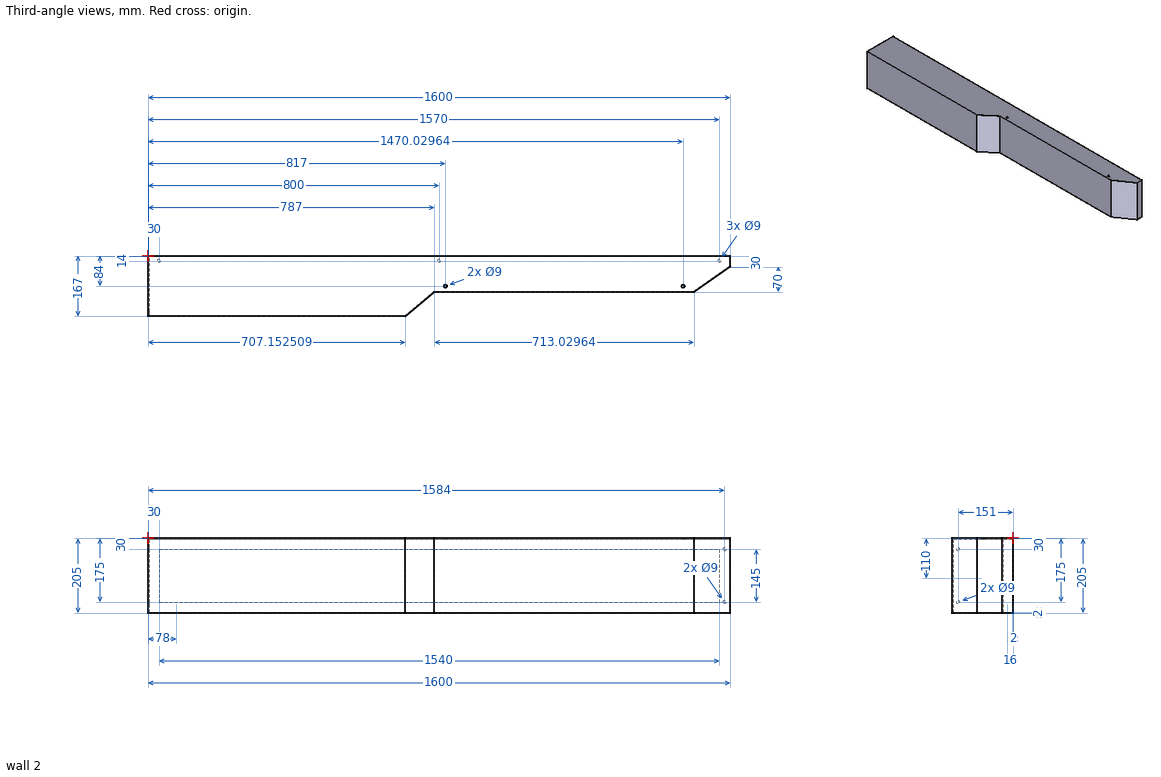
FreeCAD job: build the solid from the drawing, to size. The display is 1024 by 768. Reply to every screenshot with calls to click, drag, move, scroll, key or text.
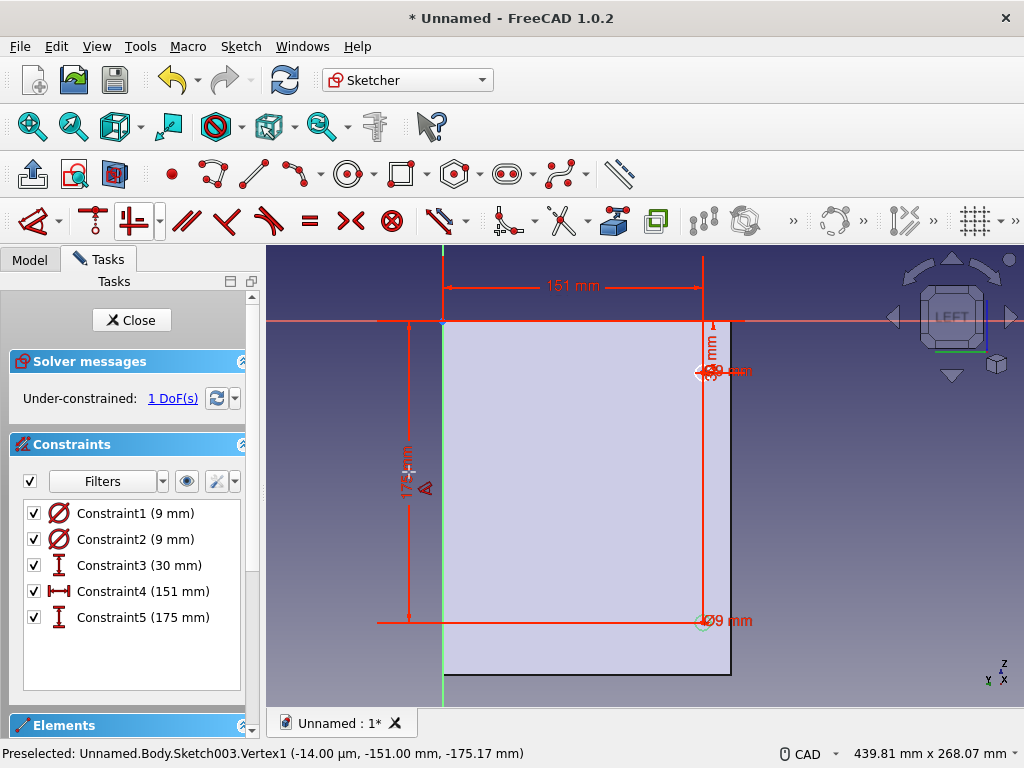
click(703, 373)
click(482, 287)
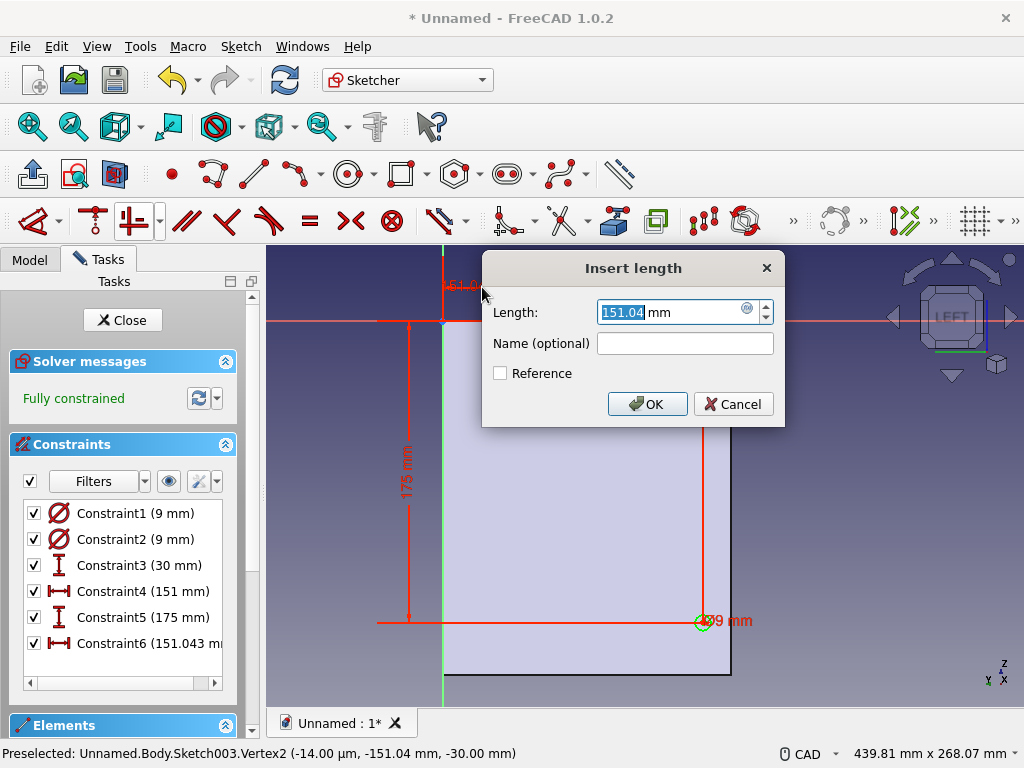
text(151)
key(Return)
key(Escape)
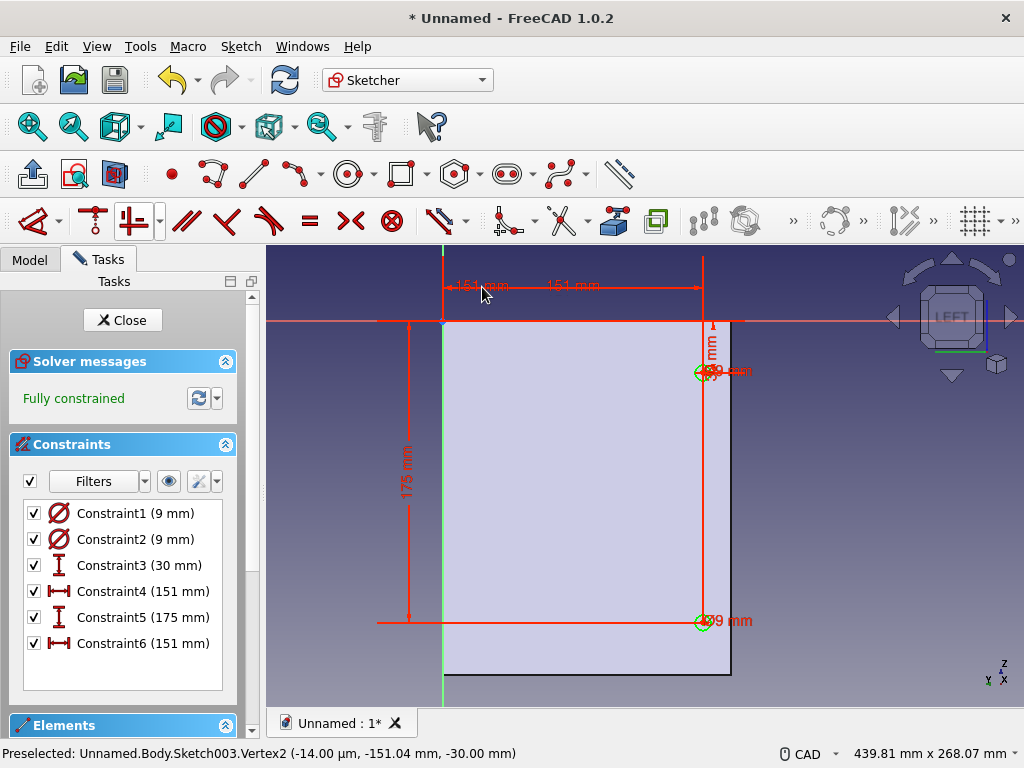
click(123, 320)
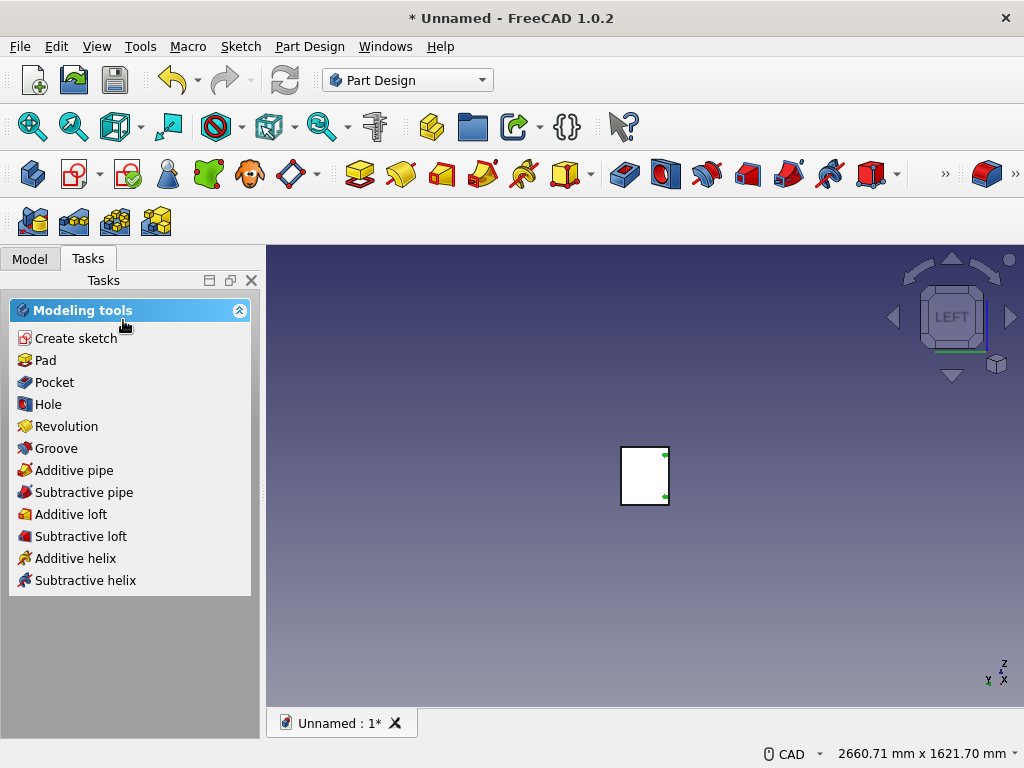
click(625, 174)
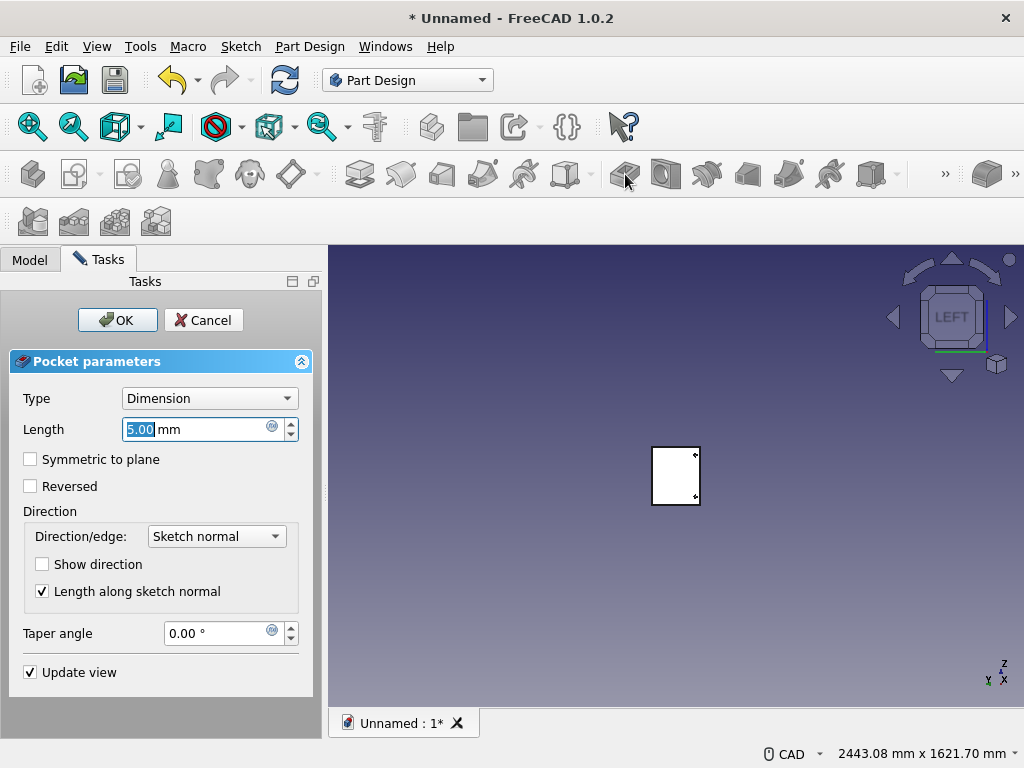
text(78)
key(Tab)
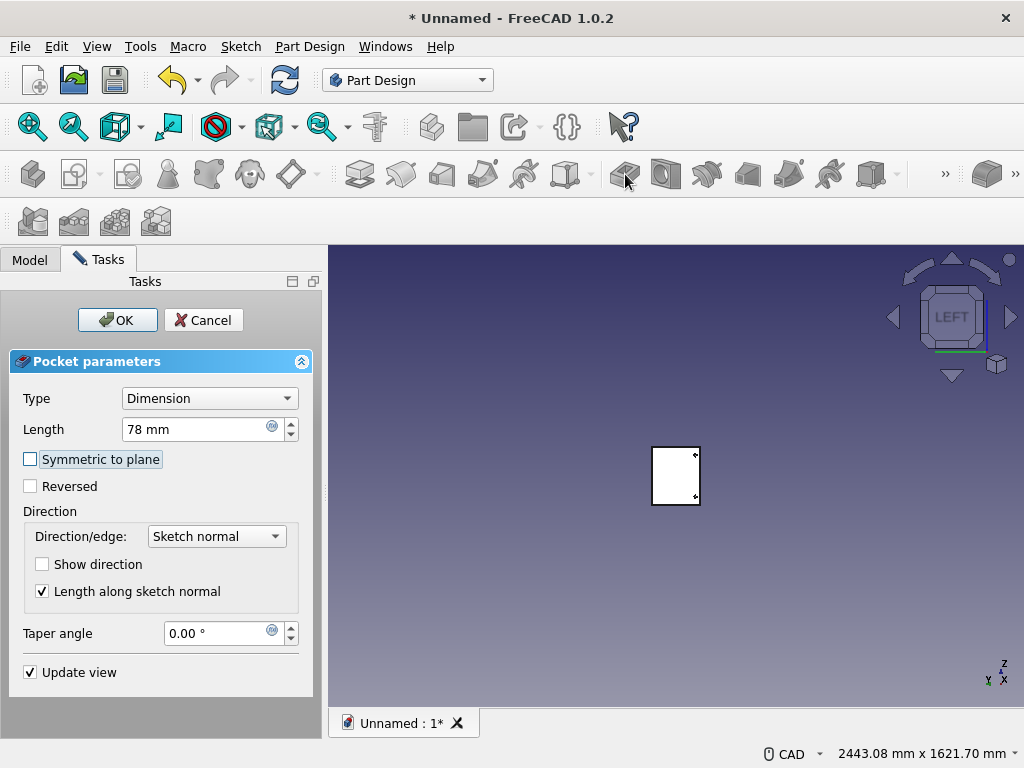
click(118, 320)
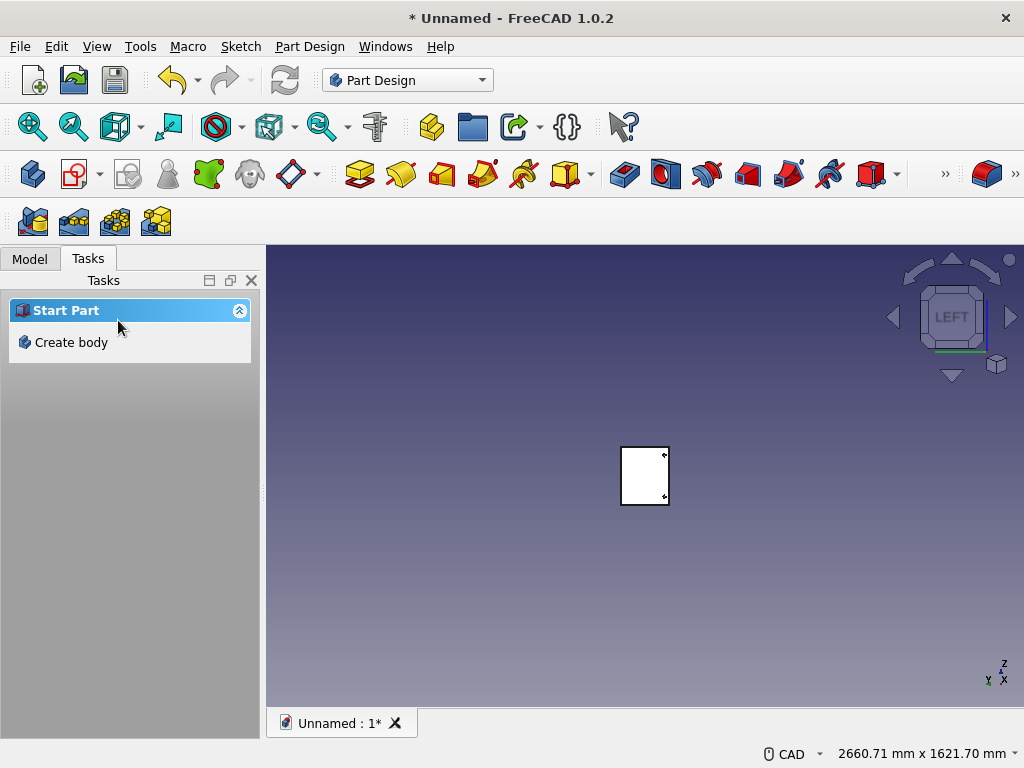
key(v)
key(f)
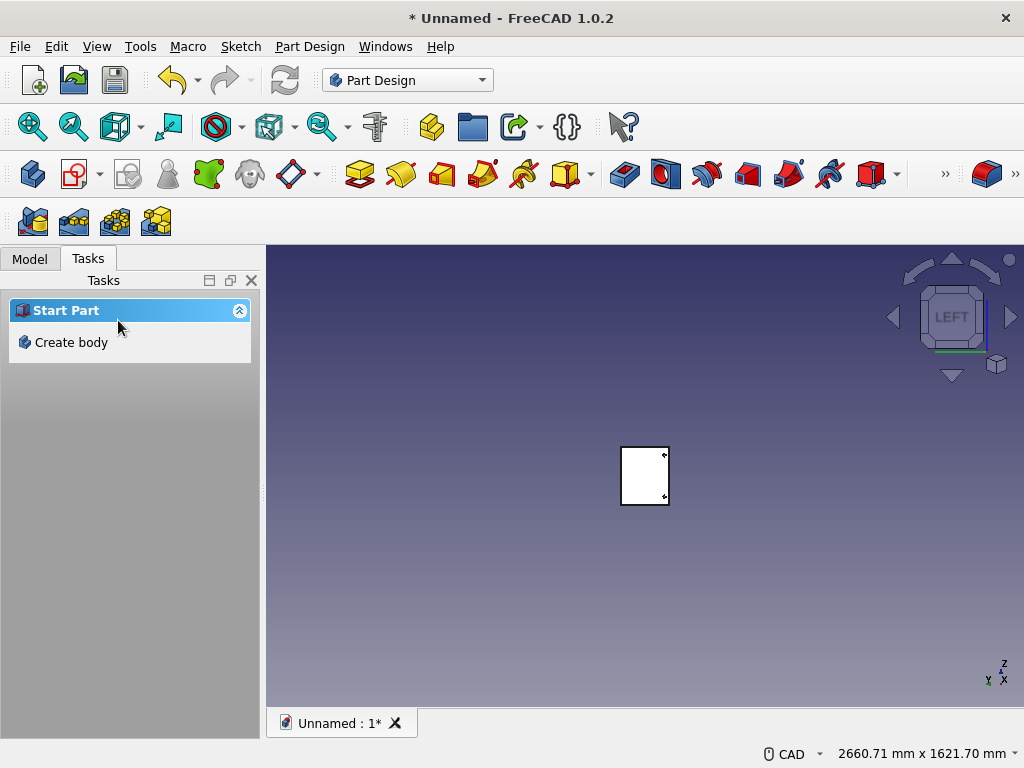
key(4)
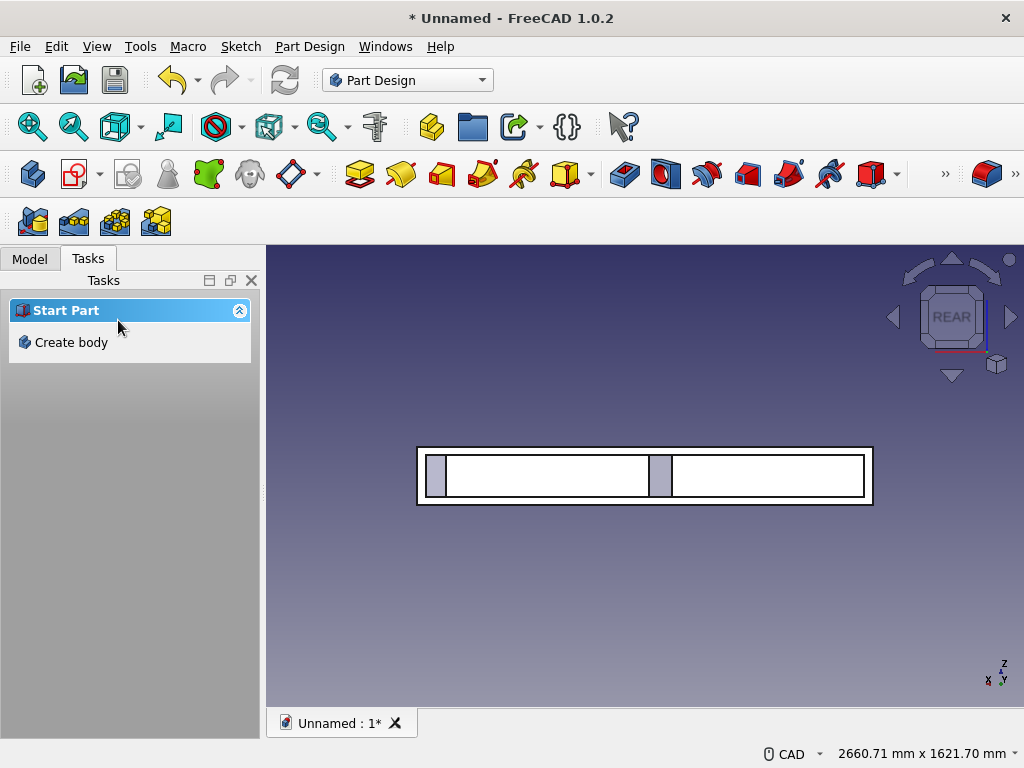
scroll(450, 450, up, 6)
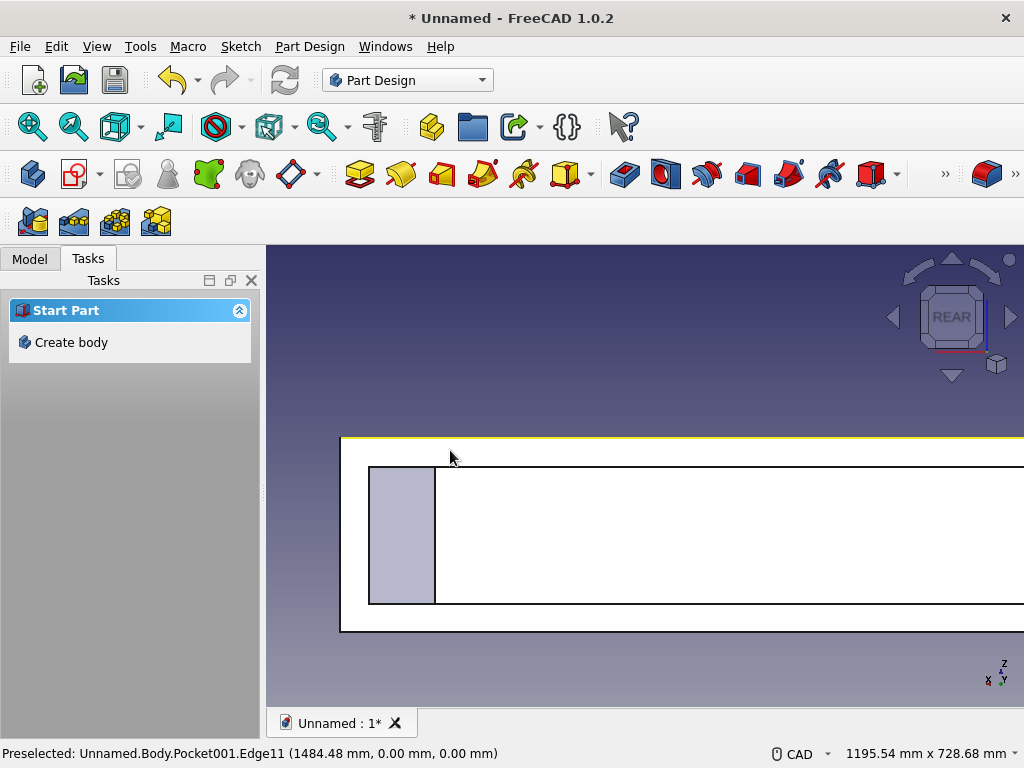
click(448, 451)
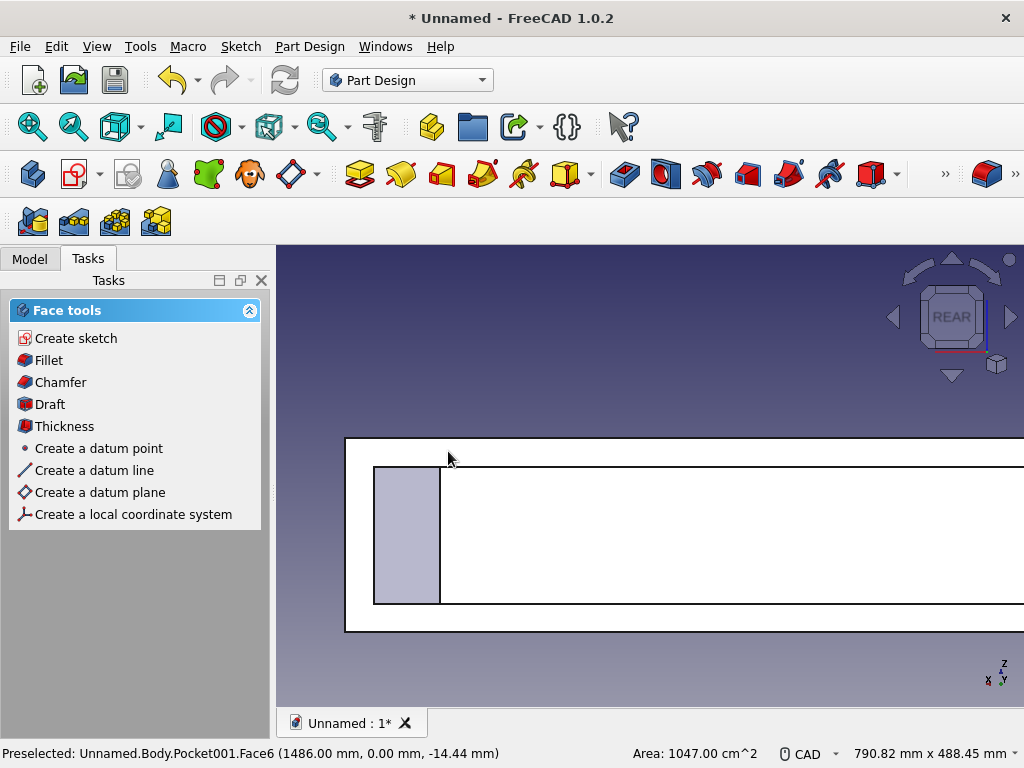
click(74, 174)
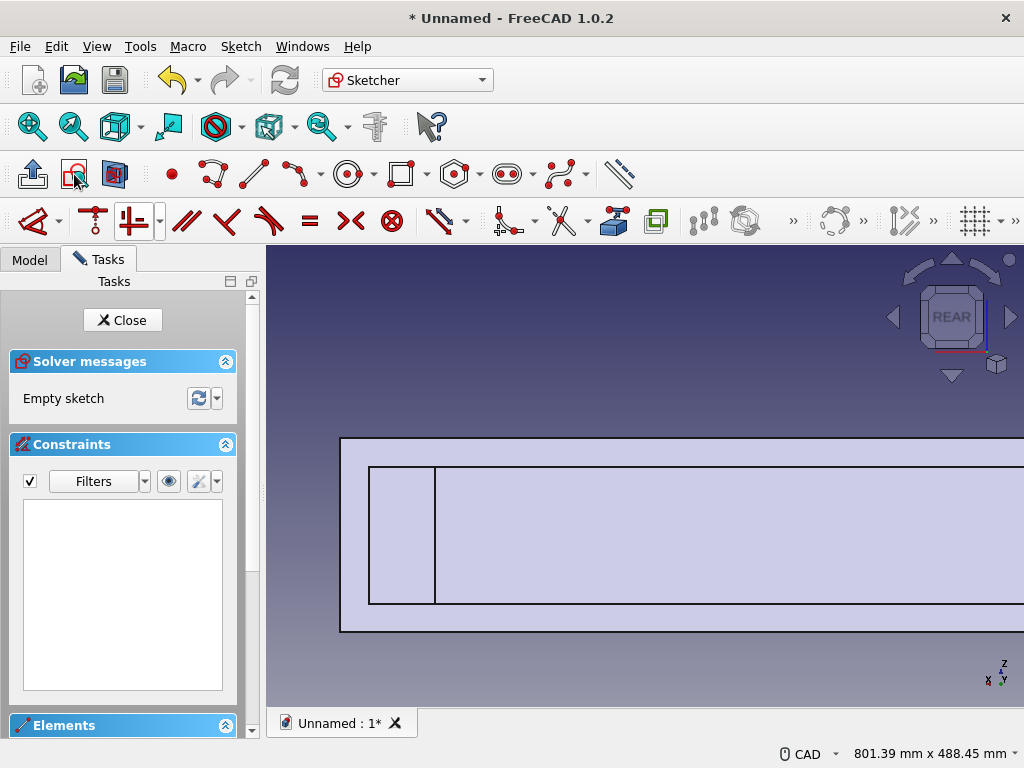
scroll(294, 607, up, 3)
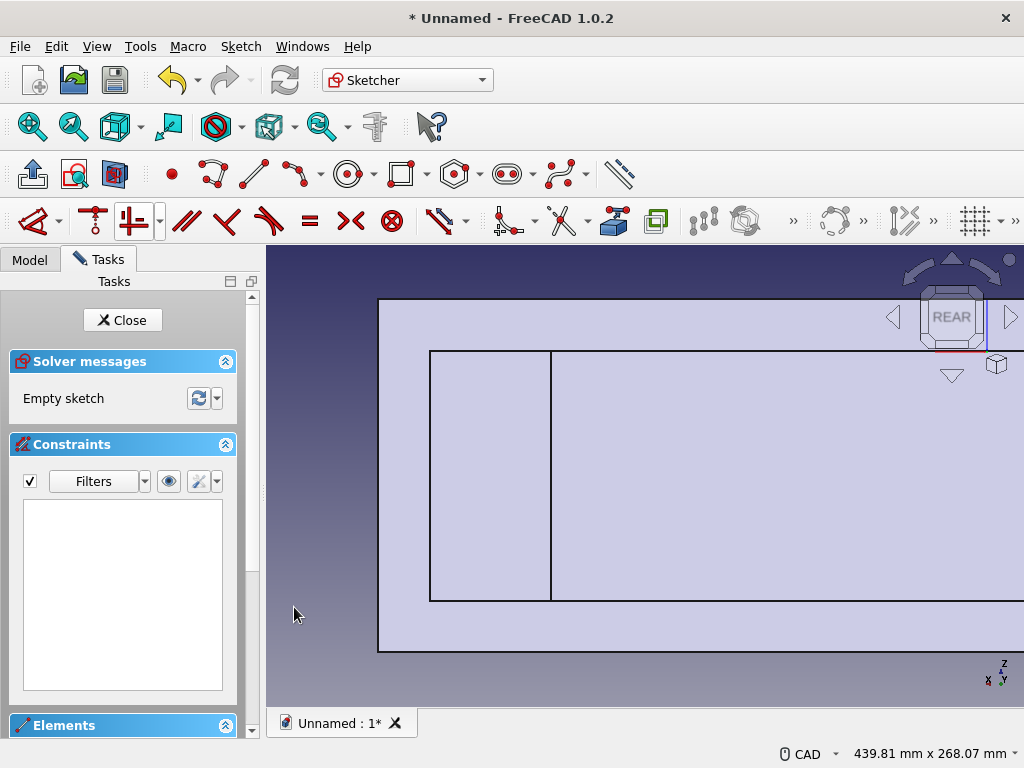
click(348, 174)